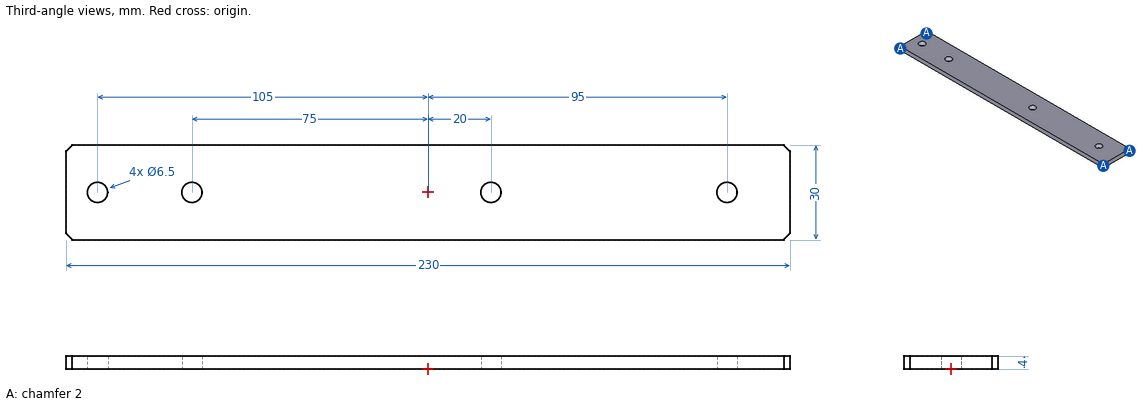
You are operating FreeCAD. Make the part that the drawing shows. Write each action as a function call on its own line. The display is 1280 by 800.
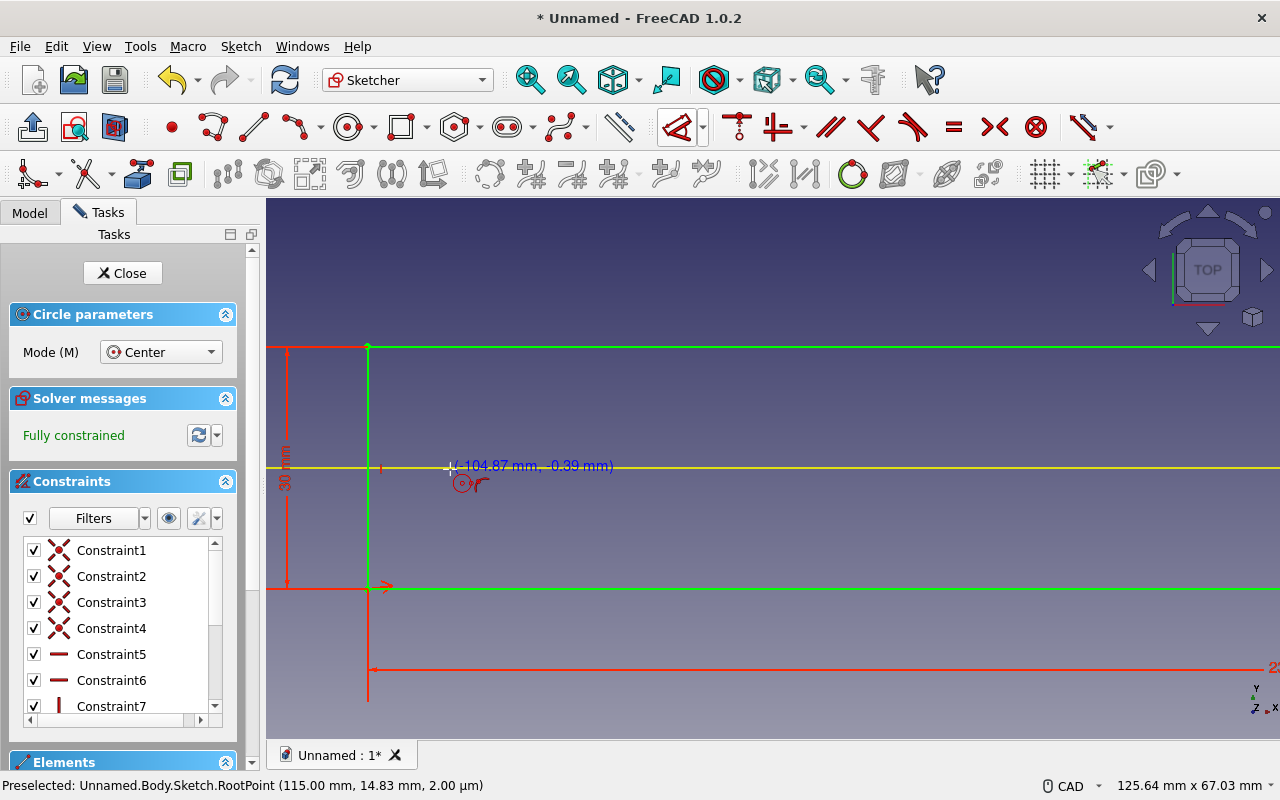
click(449, 468)
move(467, 449)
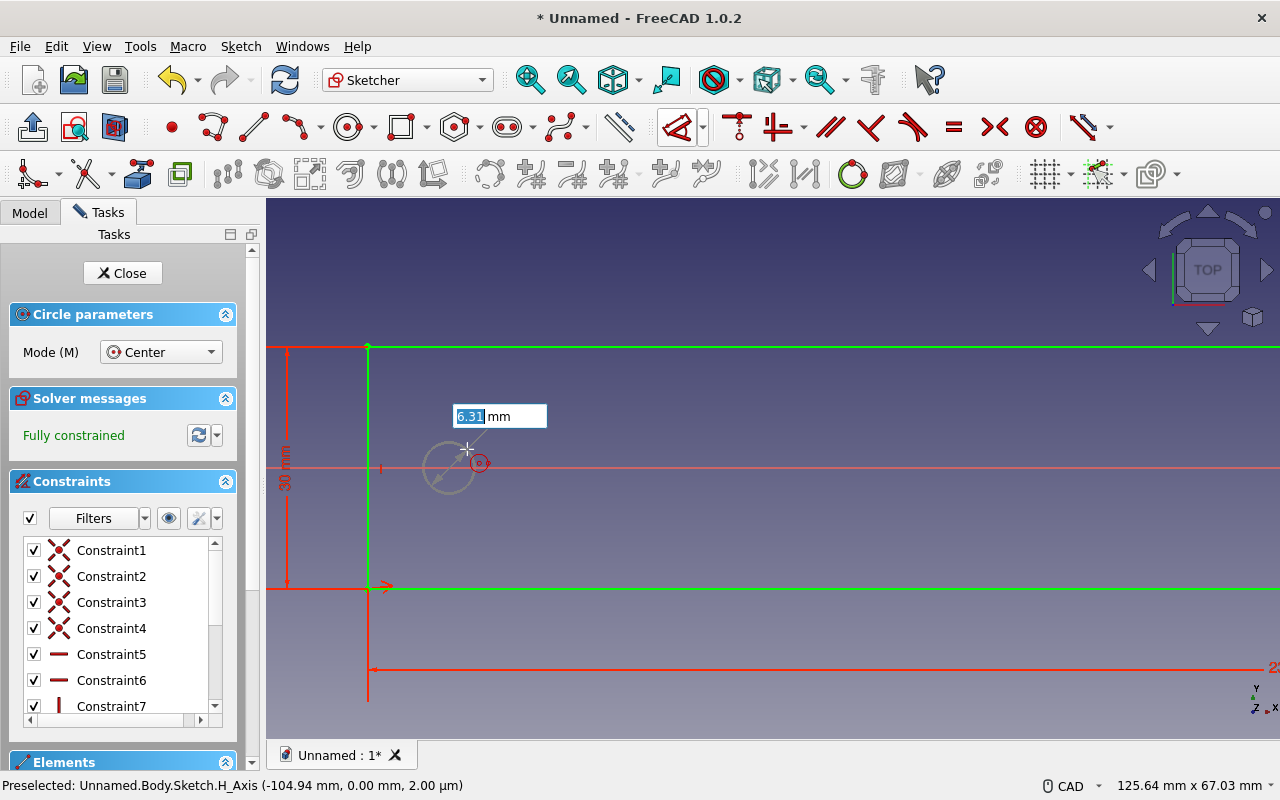
text(6.5)
key(Return)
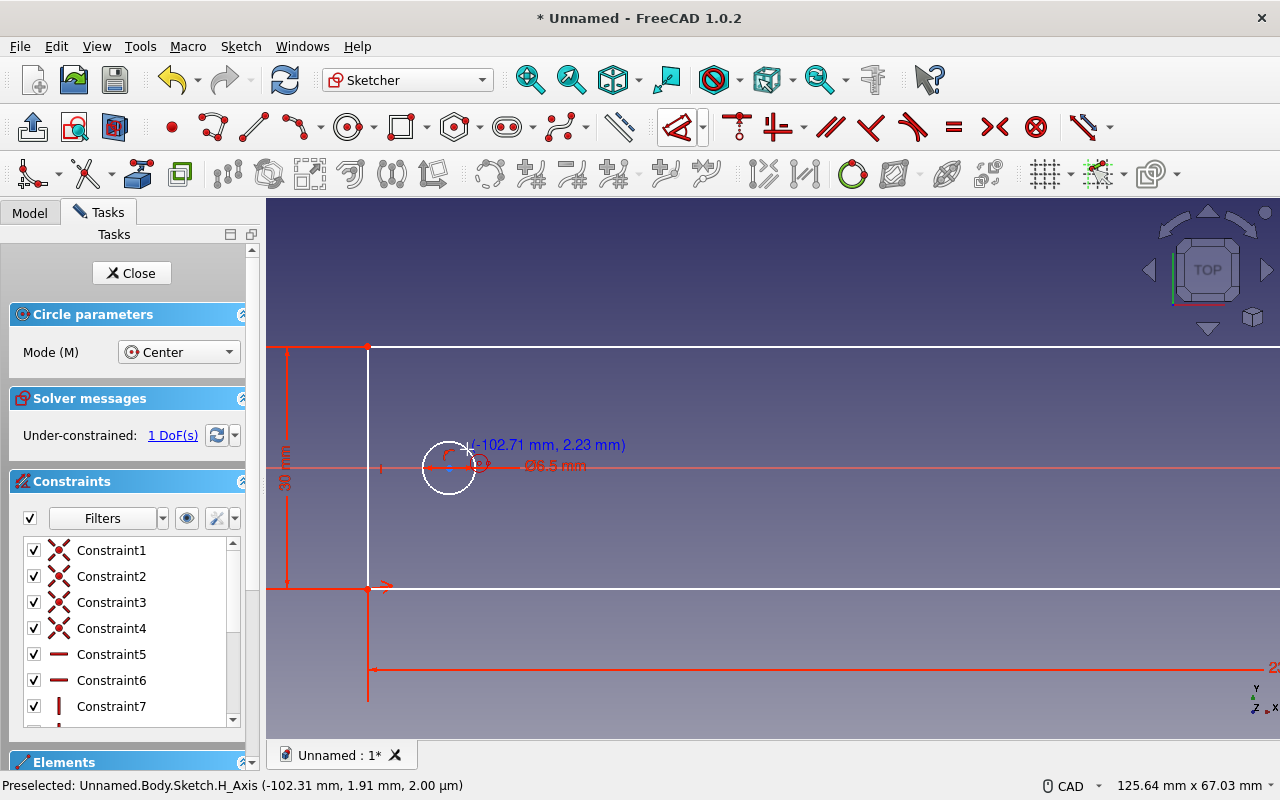
click(691, 468)
move(709, 449)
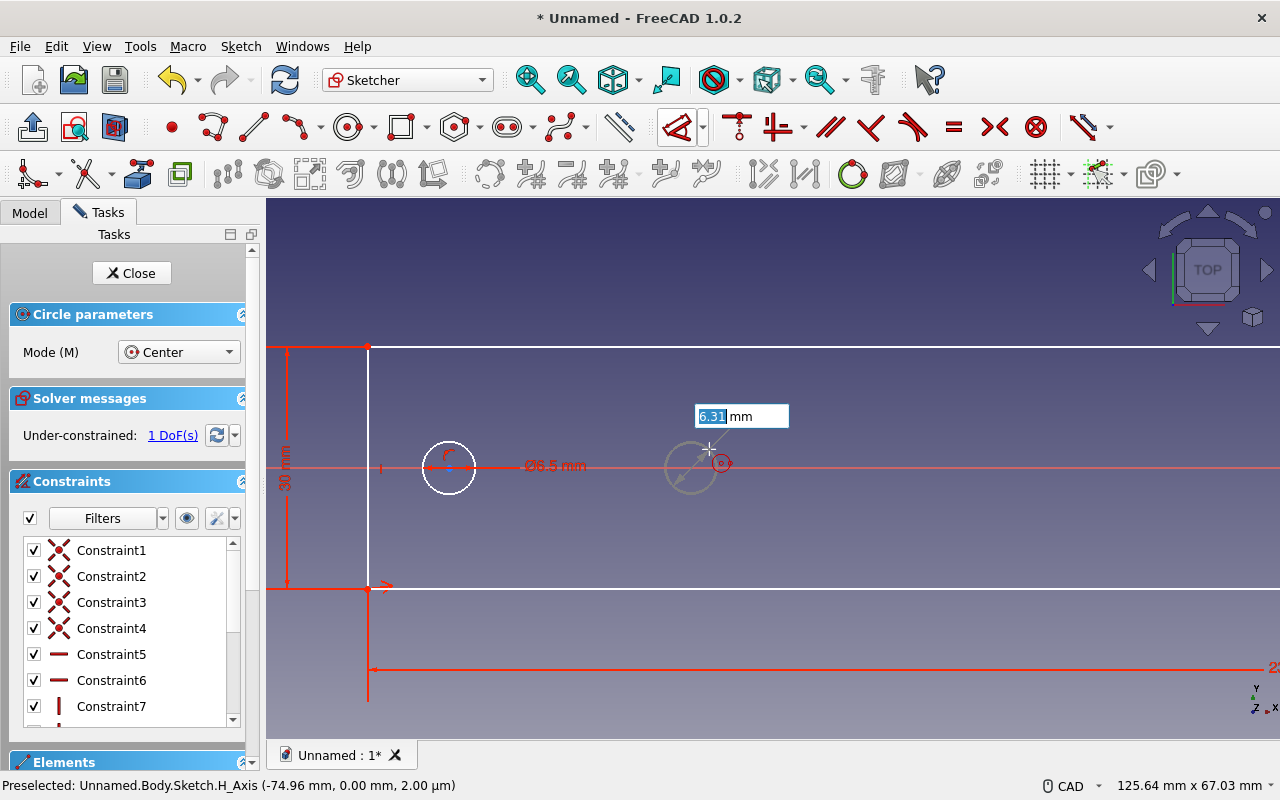
text(6.5)
key(Return)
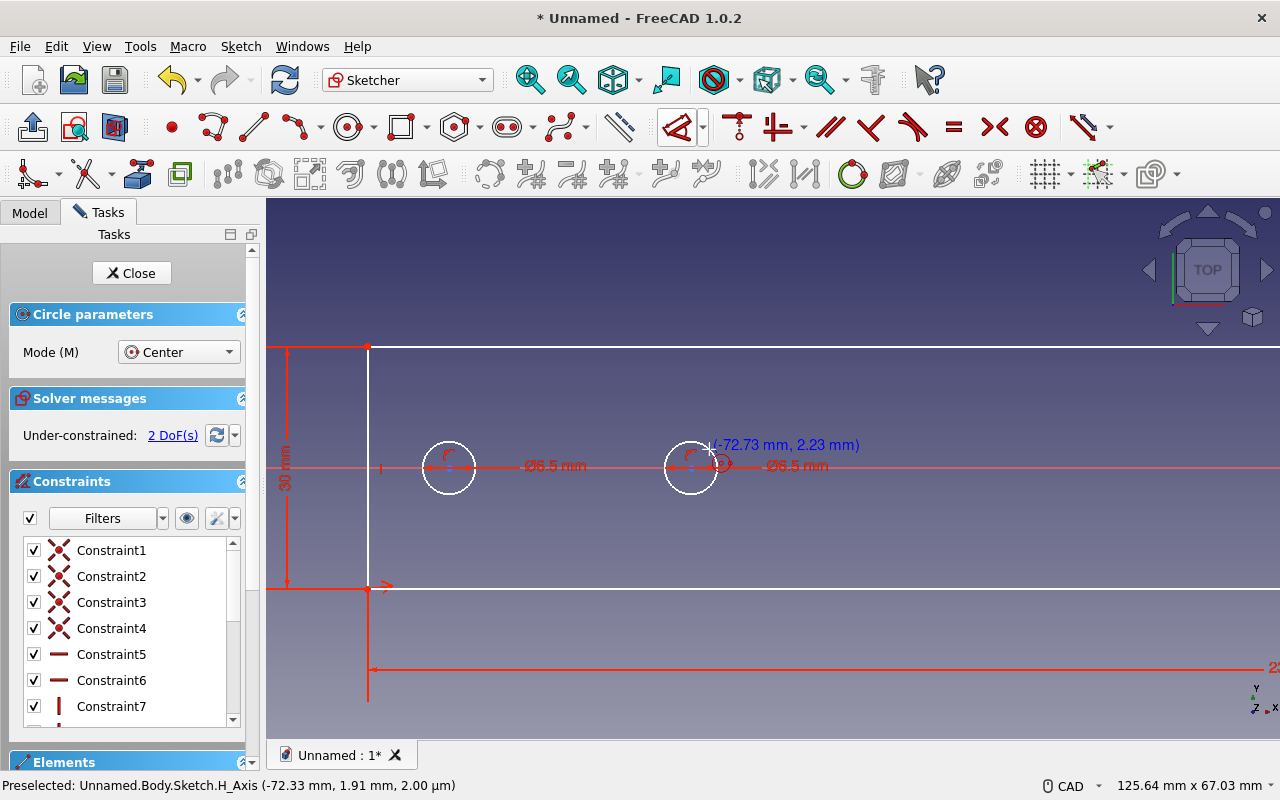
scroll(450, 469, down, 6)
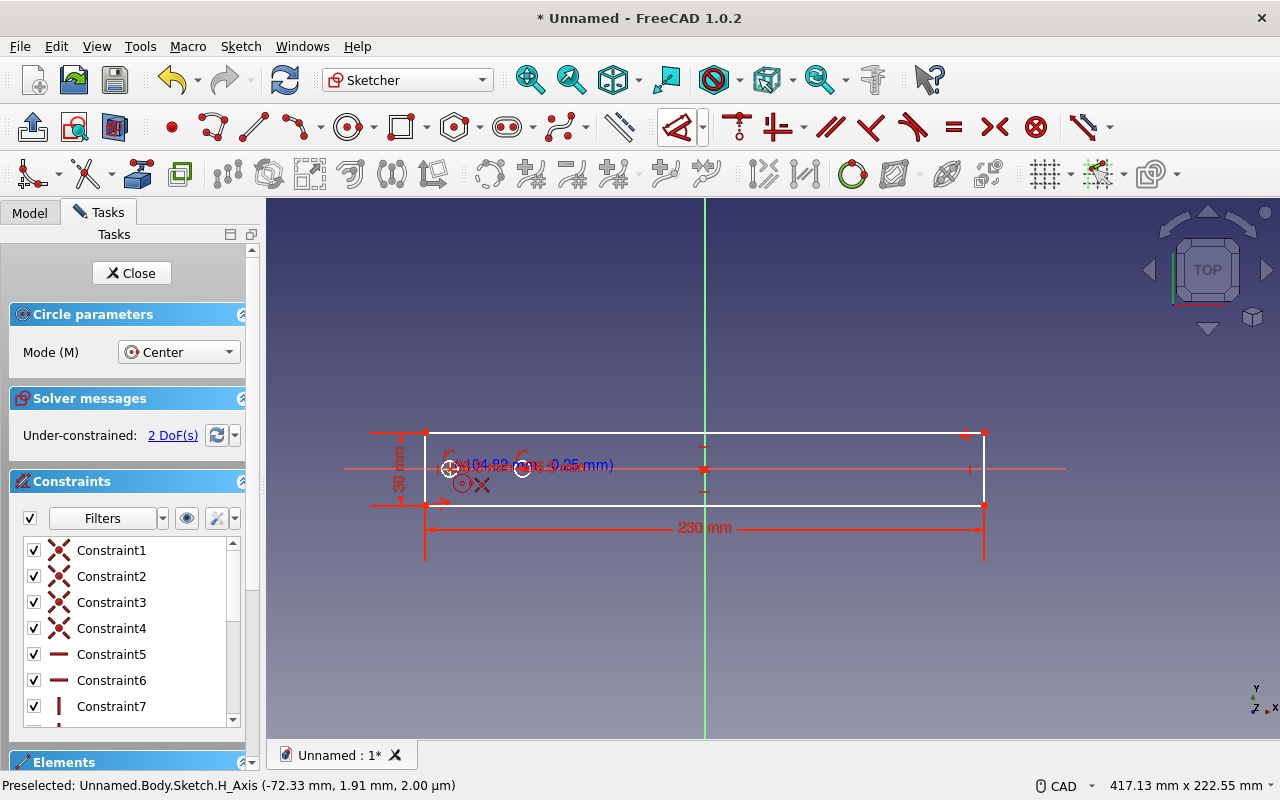
scroll(754, 469, up, 6)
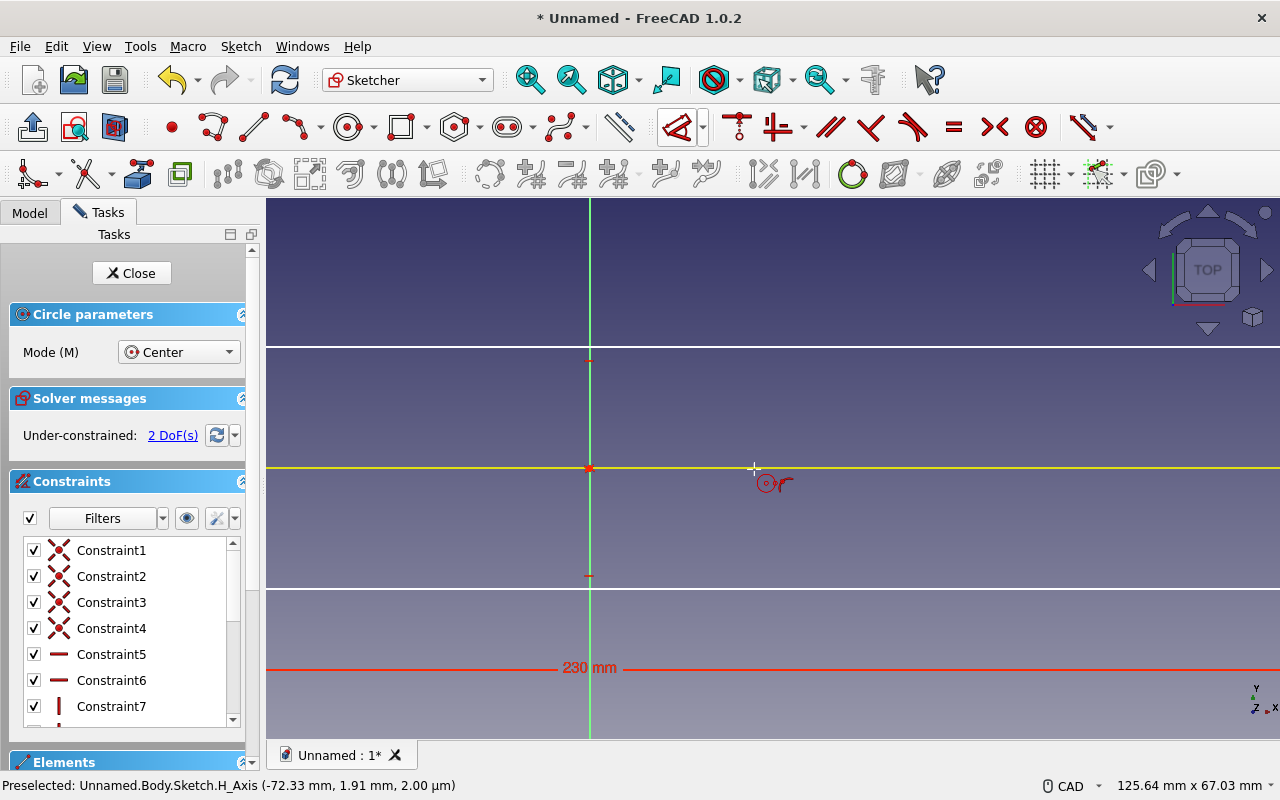
click(751, 468)
move(770, 449)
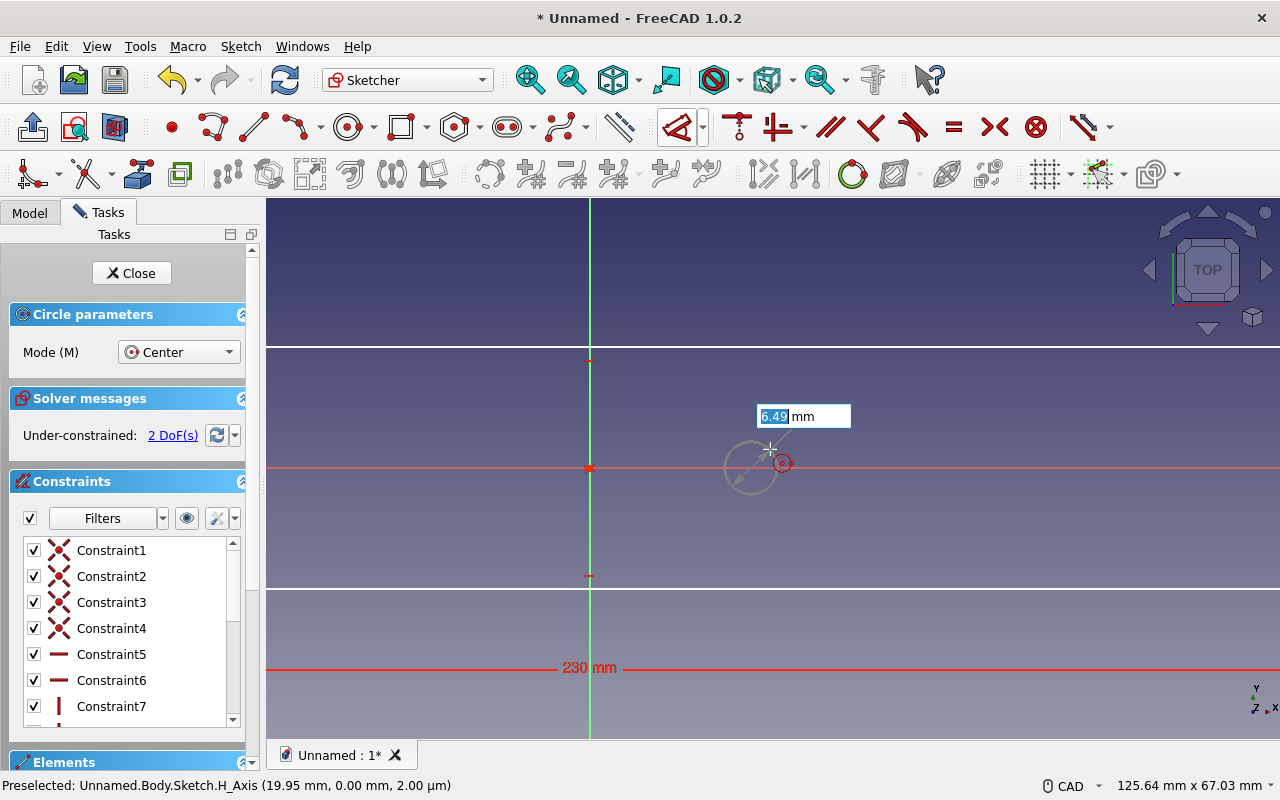
text(6.5)
key(Return)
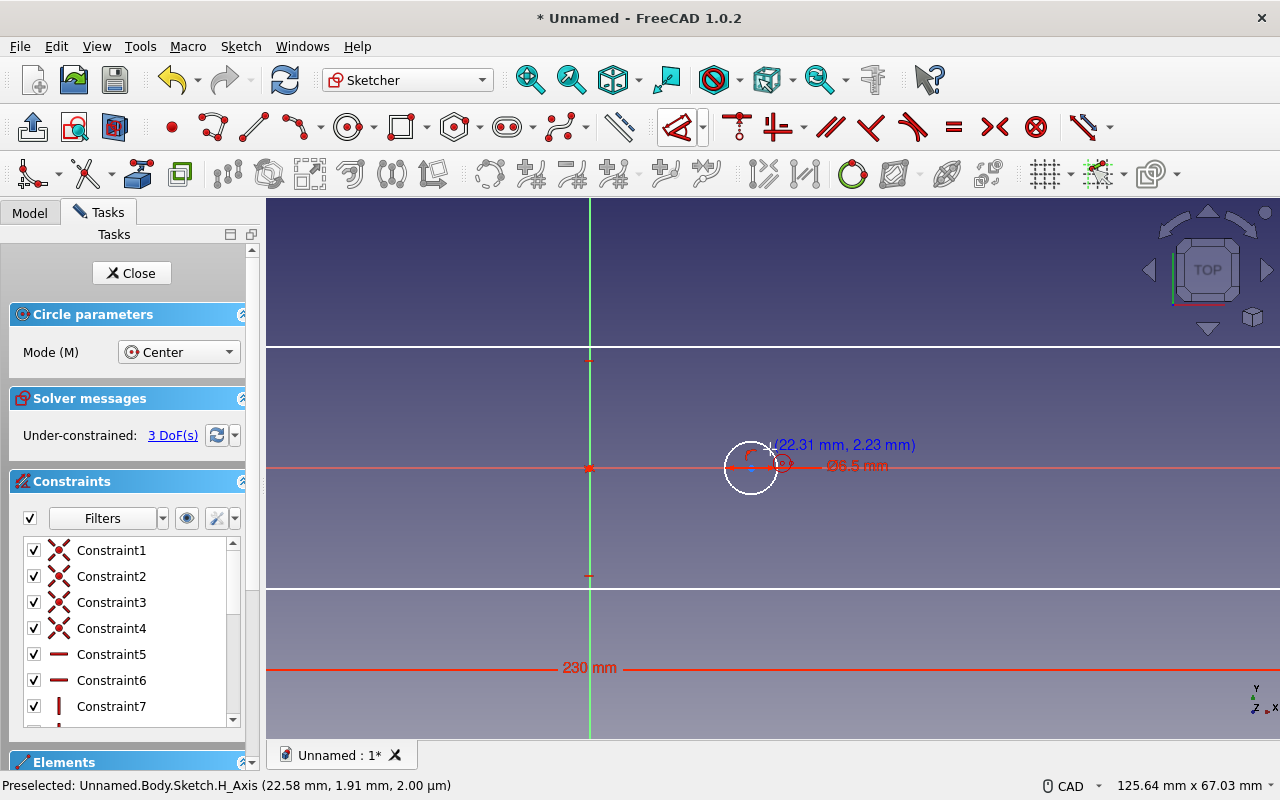
scroll(754, 469, down, 6)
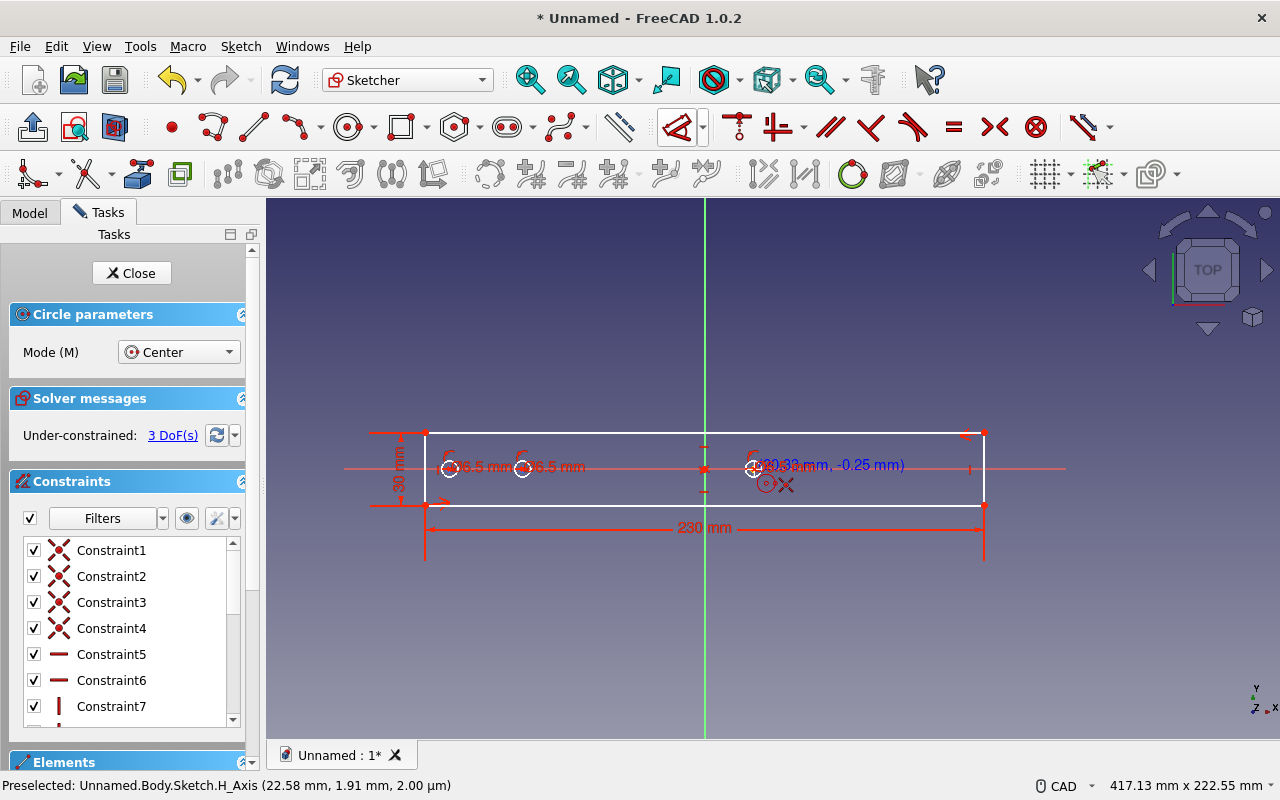
scroll(936, 469, up, 6)